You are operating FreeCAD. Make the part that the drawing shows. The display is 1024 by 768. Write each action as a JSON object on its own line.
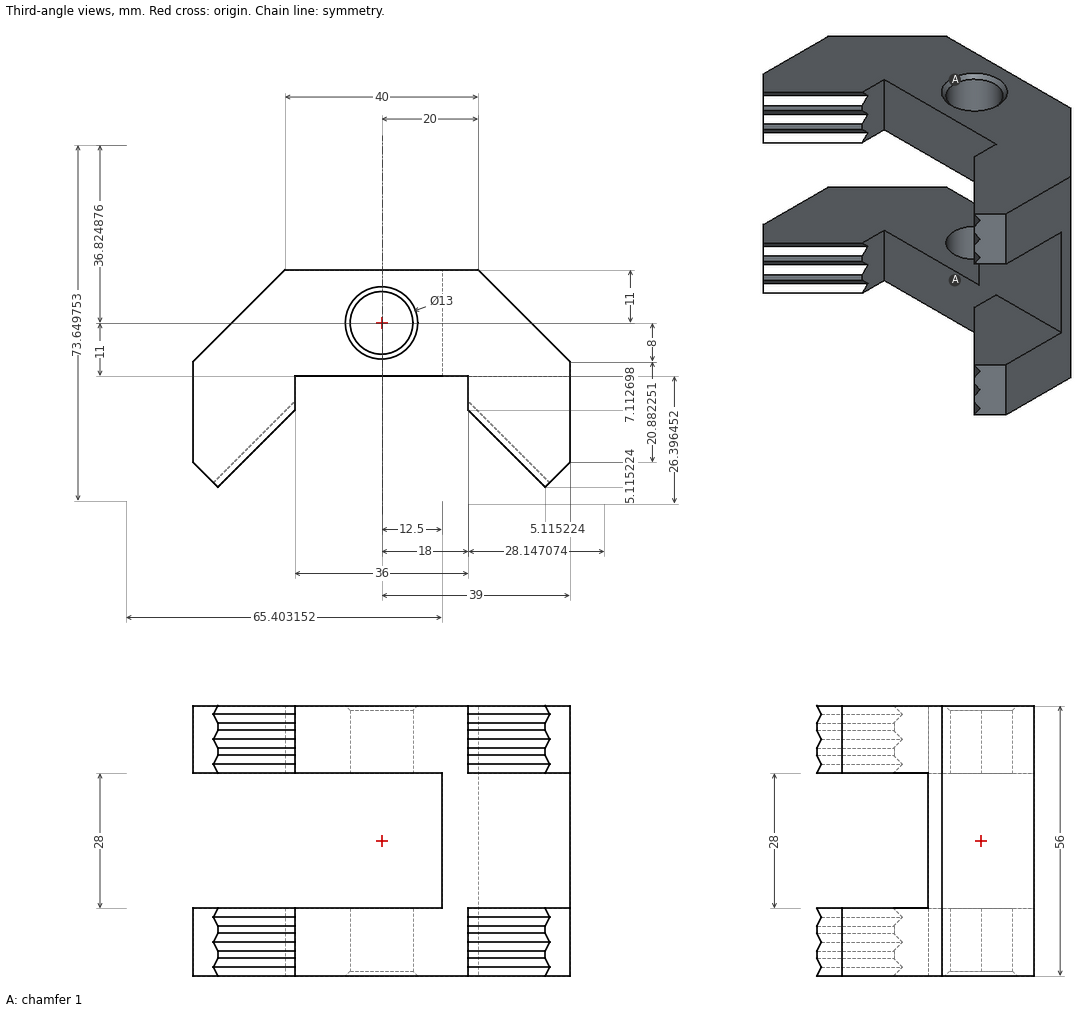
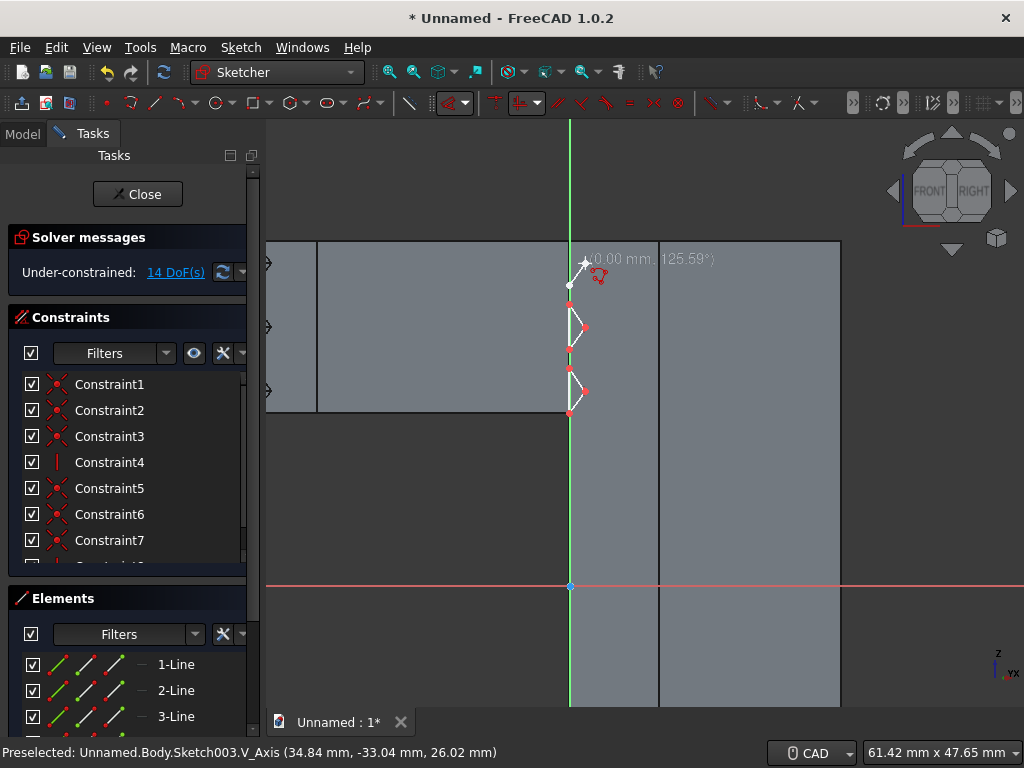
{"action": "scroll", "coordinate": [569, 241], "scroll_direction": "up", "scroll_amount": 14}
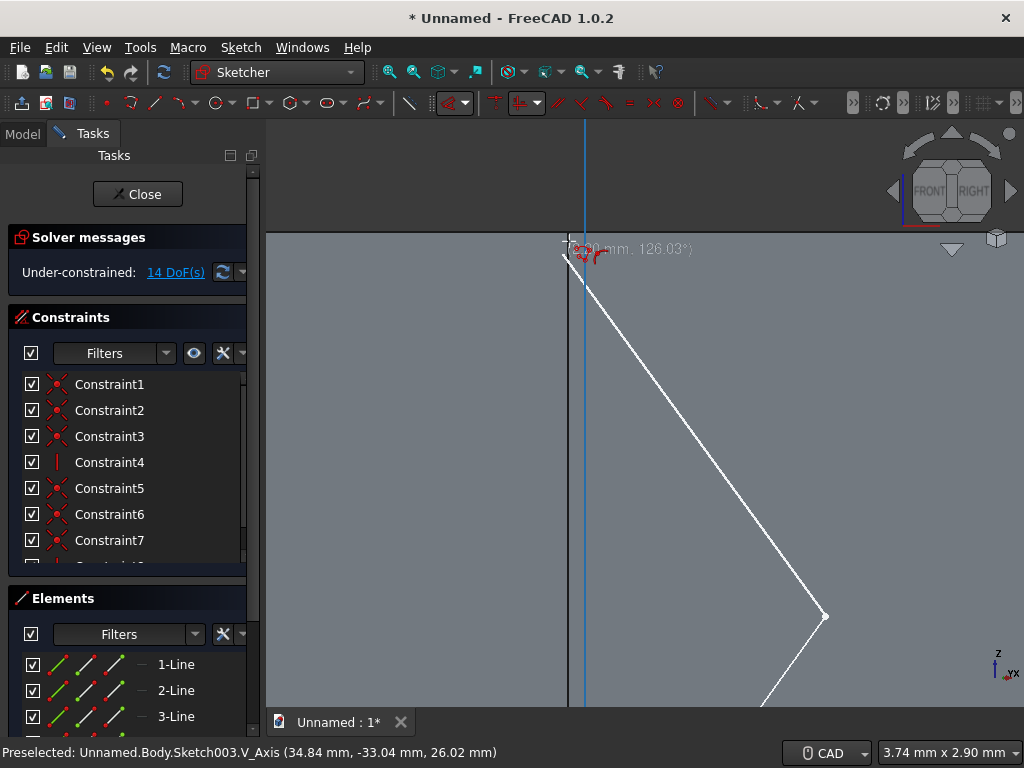
{"action": "left_click", "coordinate": [568, 232]}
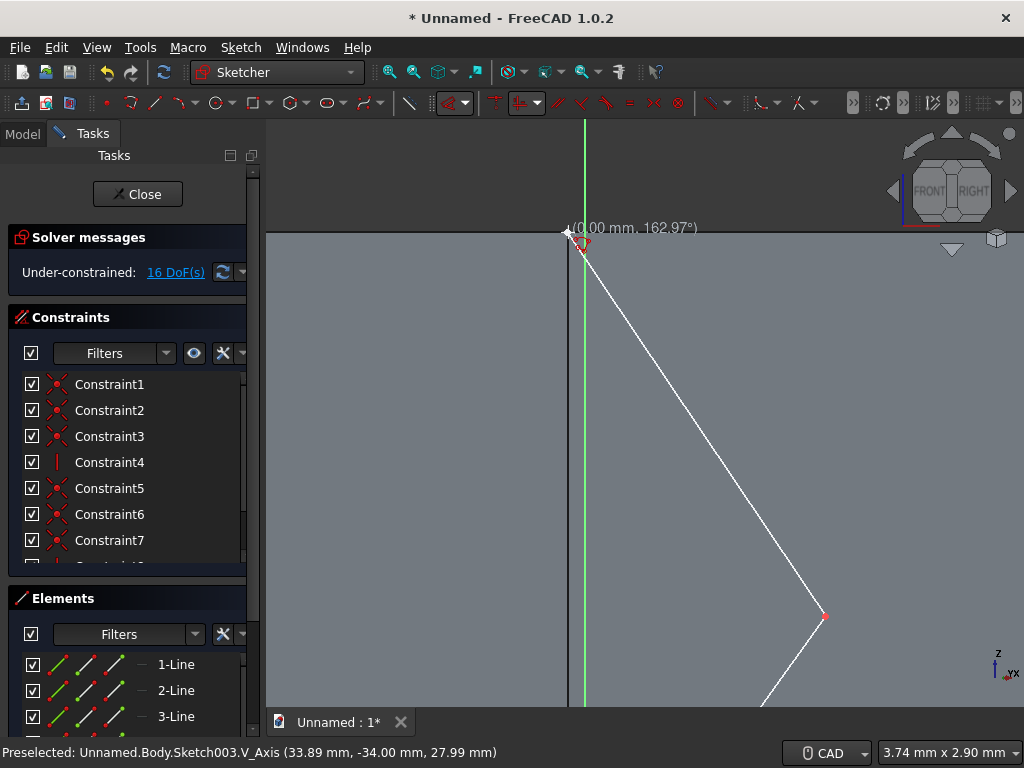
{"action": "scroll", "coordinate": [569, 241], "scroll_direction": "down", "scroll_amount": 14}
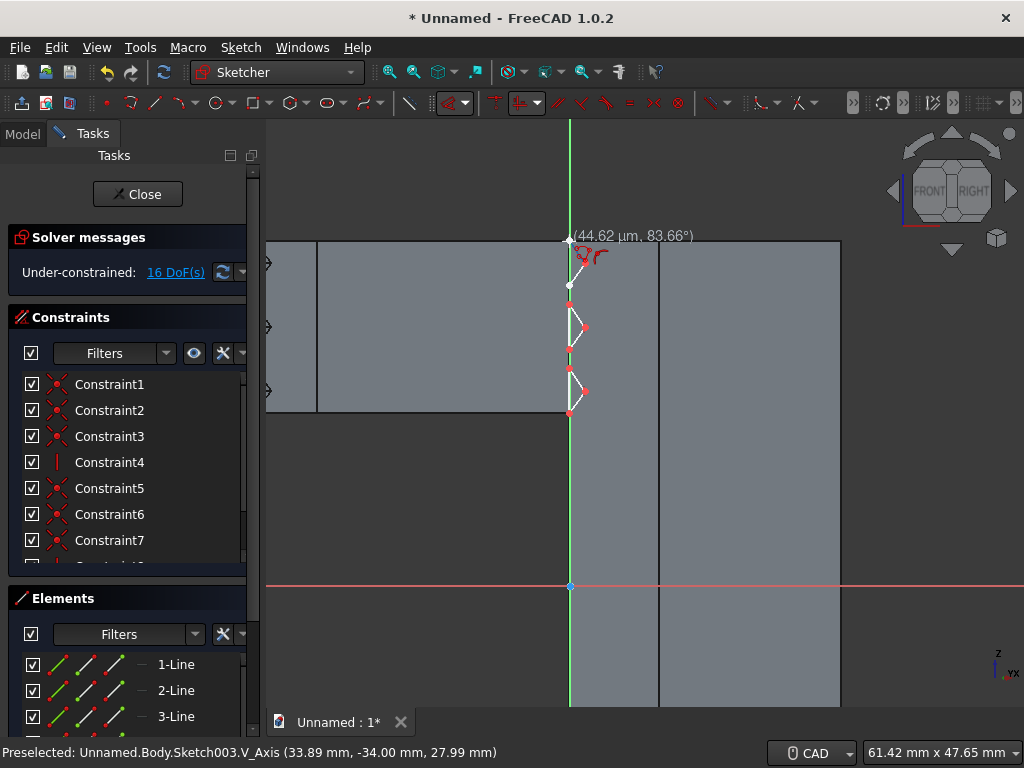
{"action": "scroll", "coordinate": [569, 286], "scroll_direction": "up", "scroll_amount": 14}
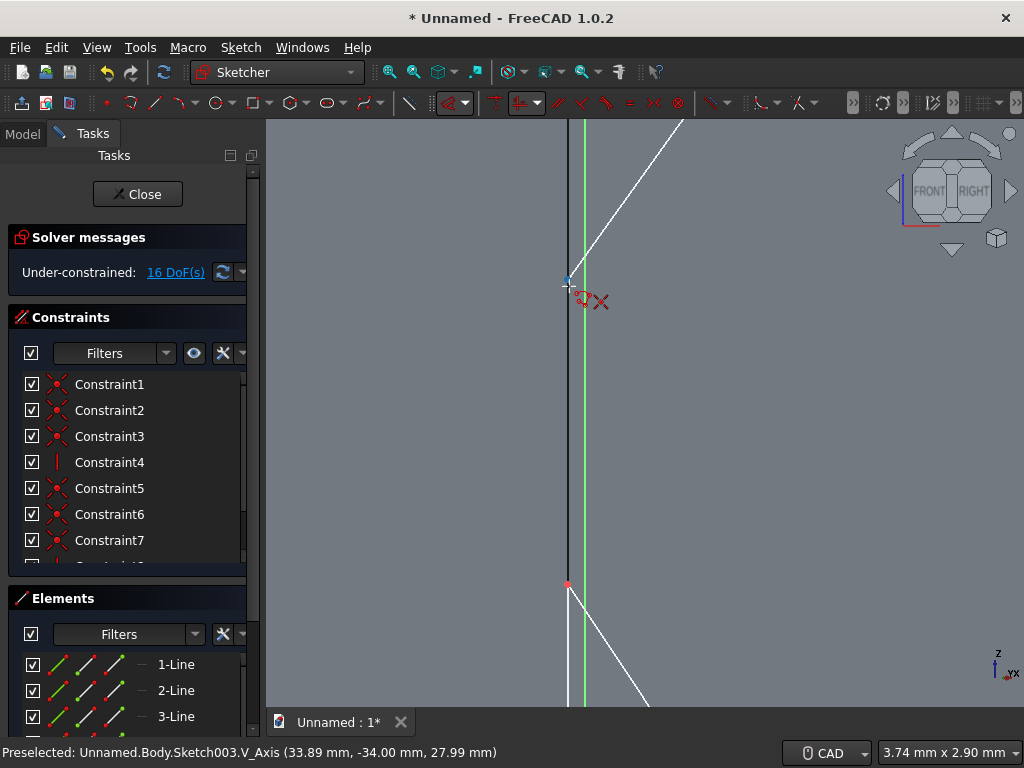
{"action": "left_click", "coordinate": [568, 280]}
{"action": "key", "text": "Escape"}
{"action": "key", "text": "Escape"}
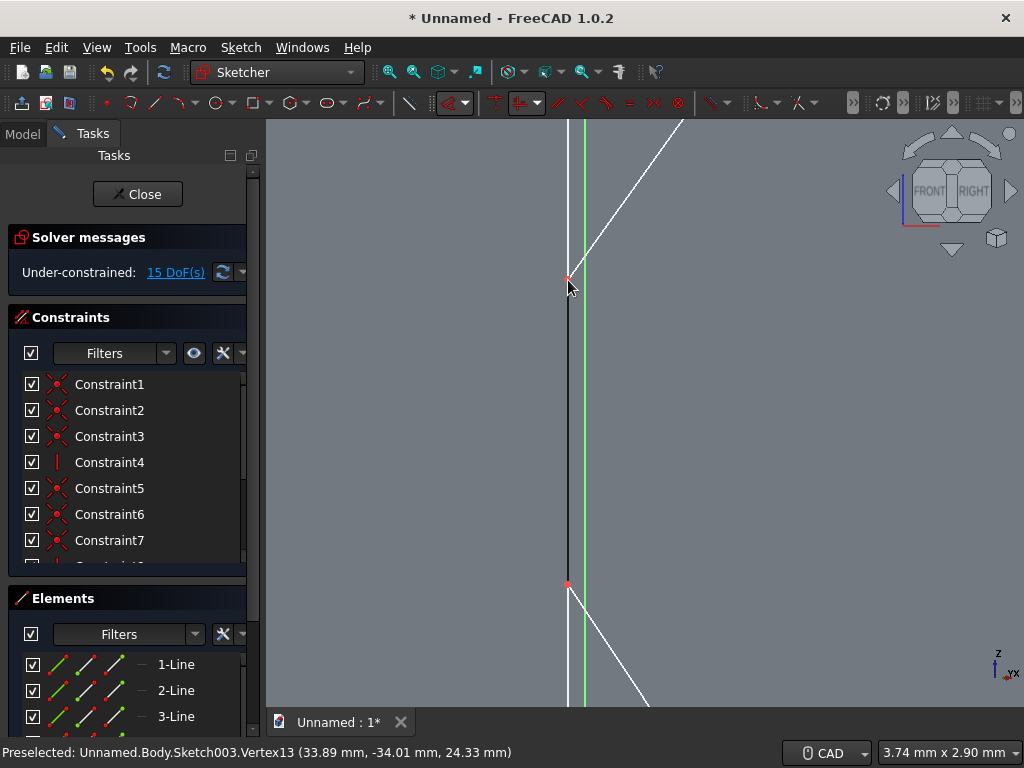
{"action": "scroll", "coordinate": [569, 286], "scroll_direction": "down", "scroll_amount": 14}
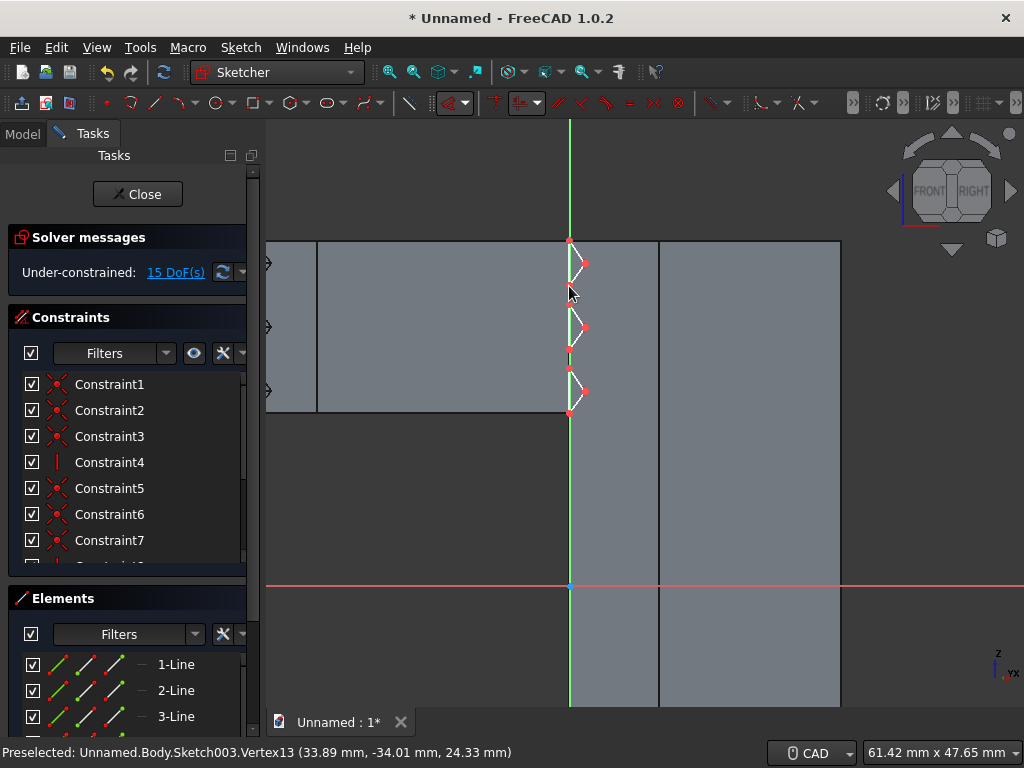
{"action": "left_click", "coordinate": [585, 328]}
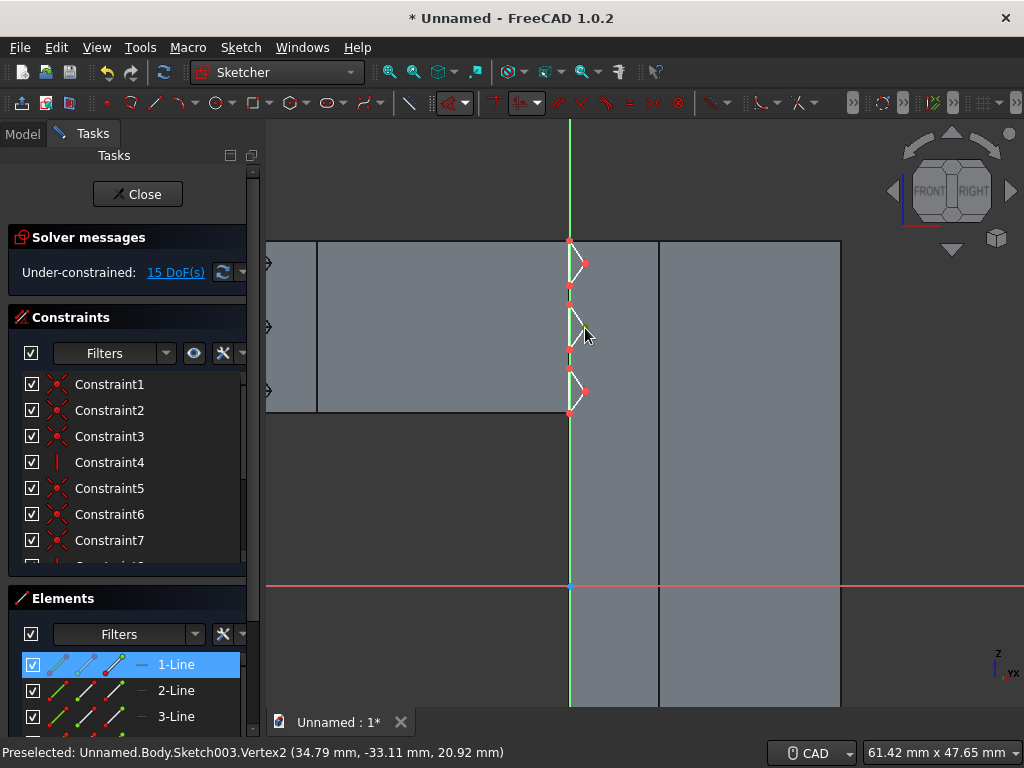
{"action": "key", "text": "i"}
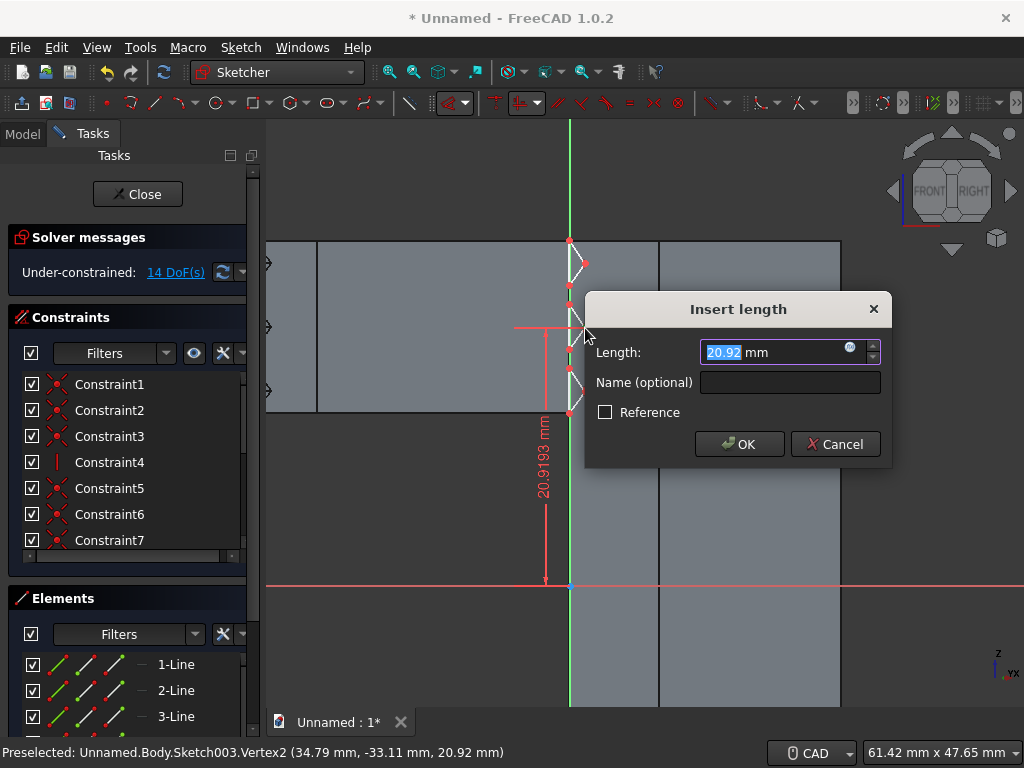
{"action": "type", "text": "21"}
{"action": "key", "text": "Return"}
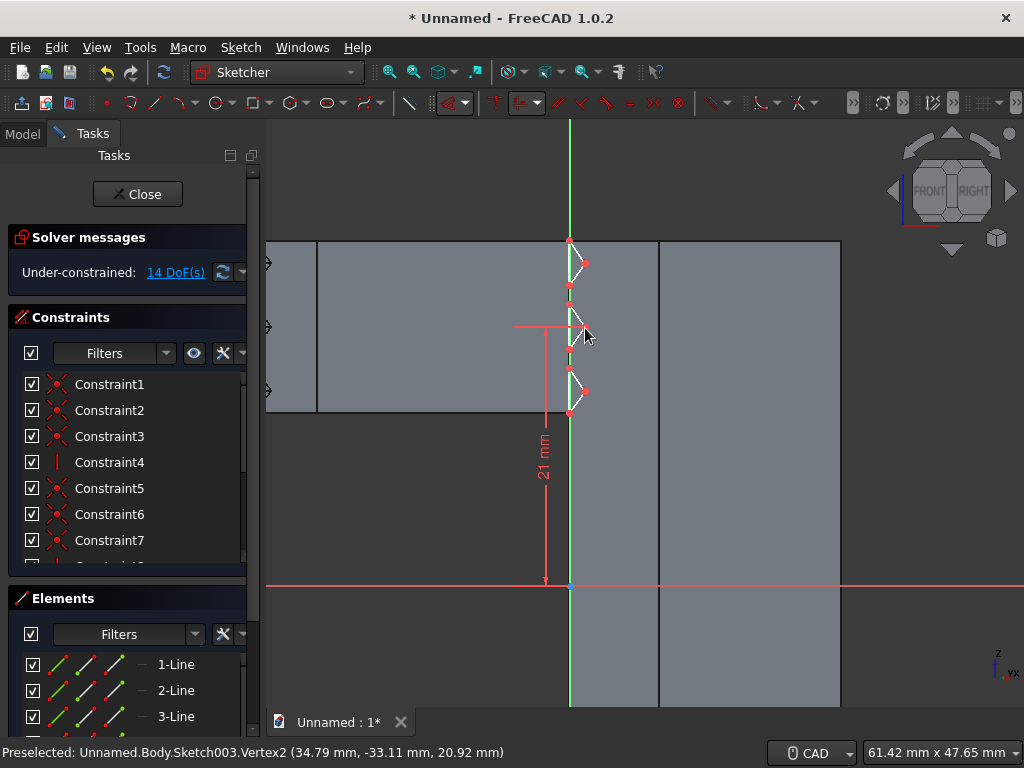
{"action": "left_click", "coordinate": [569, 413]}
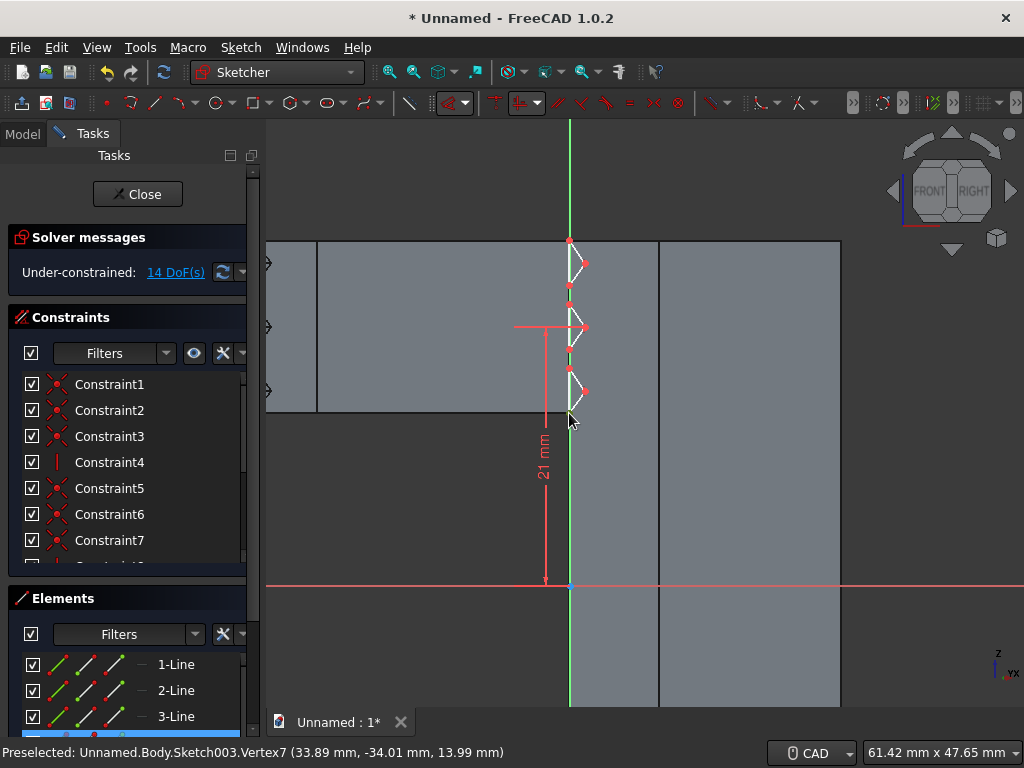
{"action": "left_click", "coordinate": [468, 104]}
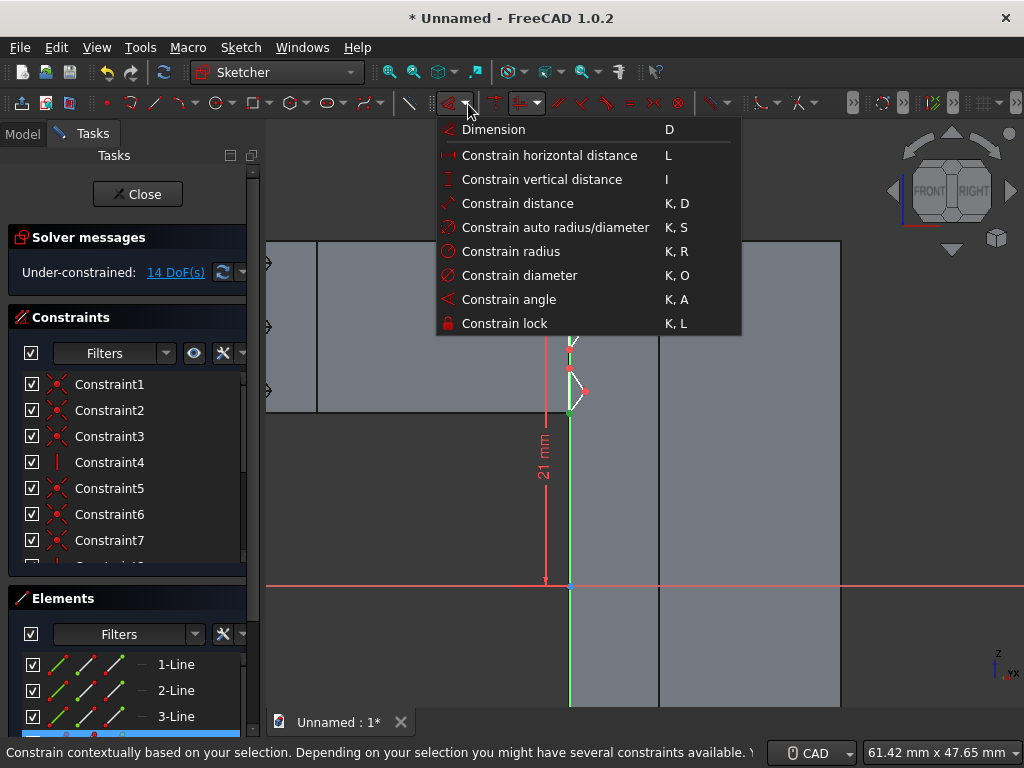
{"action": "left_click", "coordinate": [589, 179]}